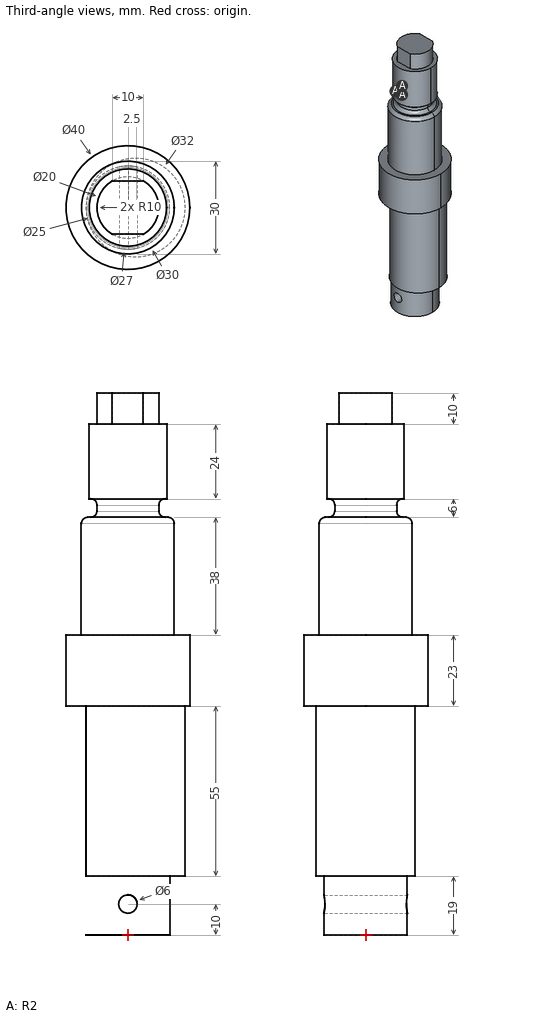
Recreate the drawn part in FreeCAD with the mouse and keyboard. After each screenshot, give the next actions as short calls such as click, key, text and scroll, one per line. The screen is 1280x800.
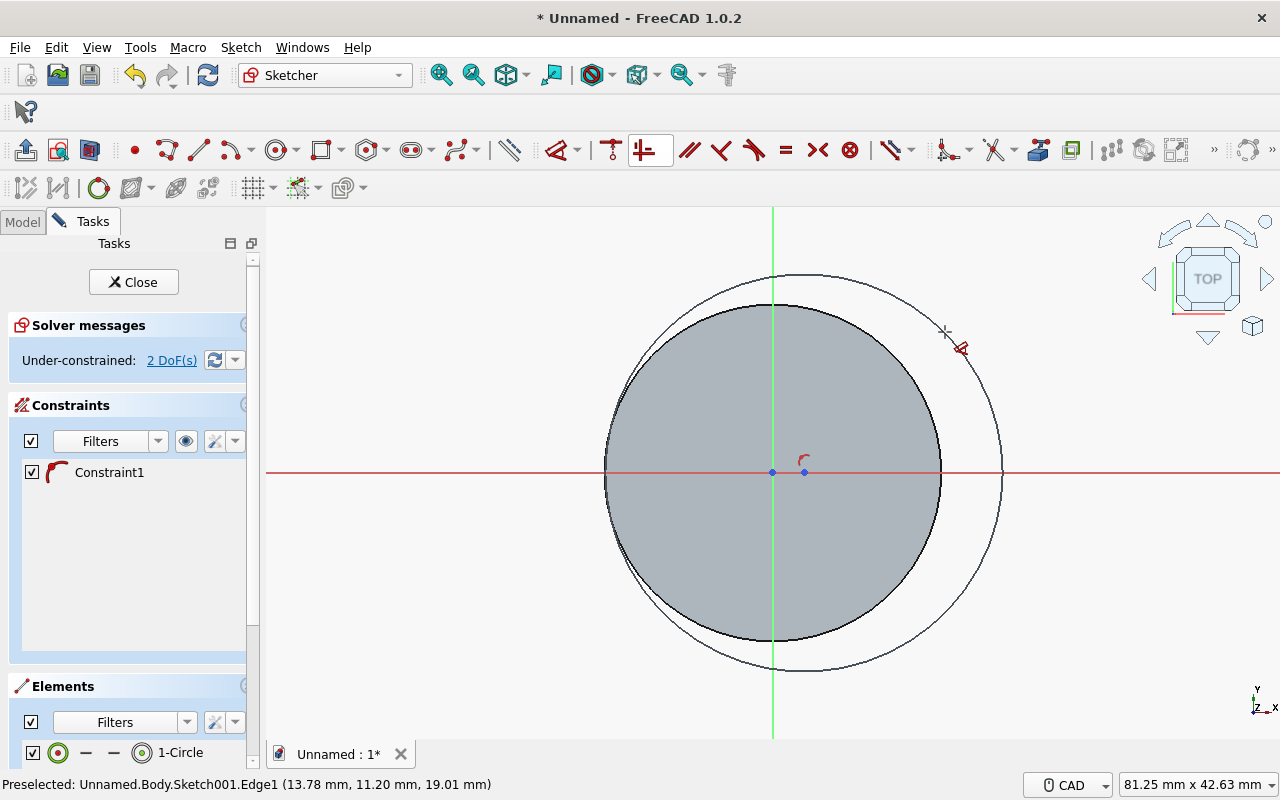
click(944, 332)
click(967, 309)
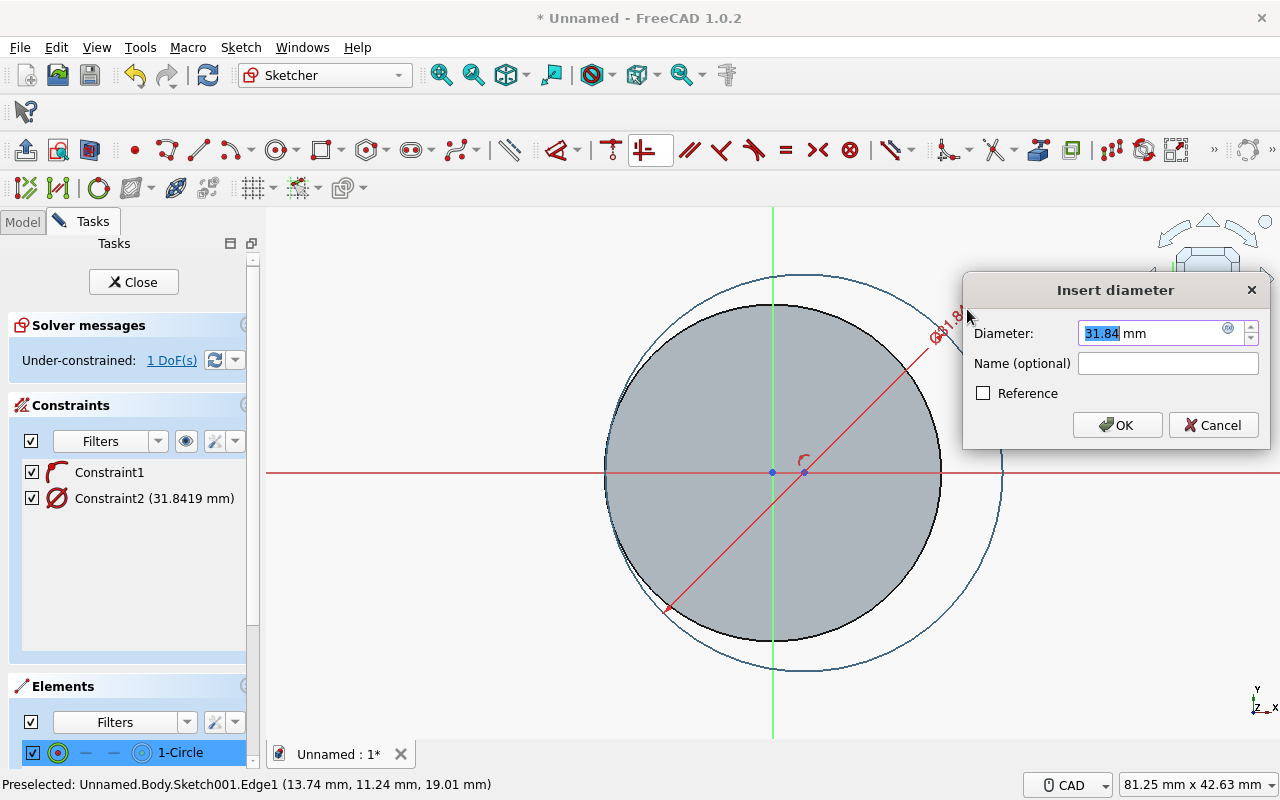
text(32)
key(Return)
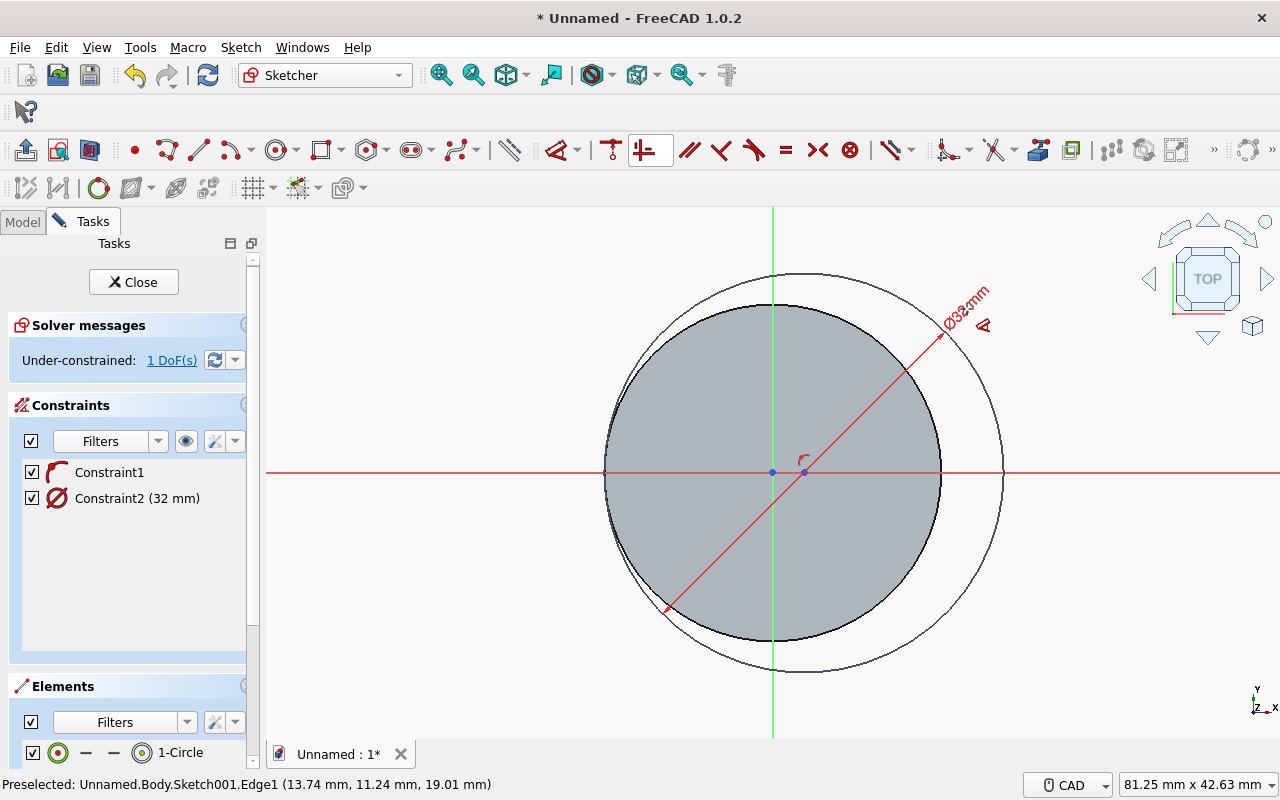
scroll(804, 473, up, 2)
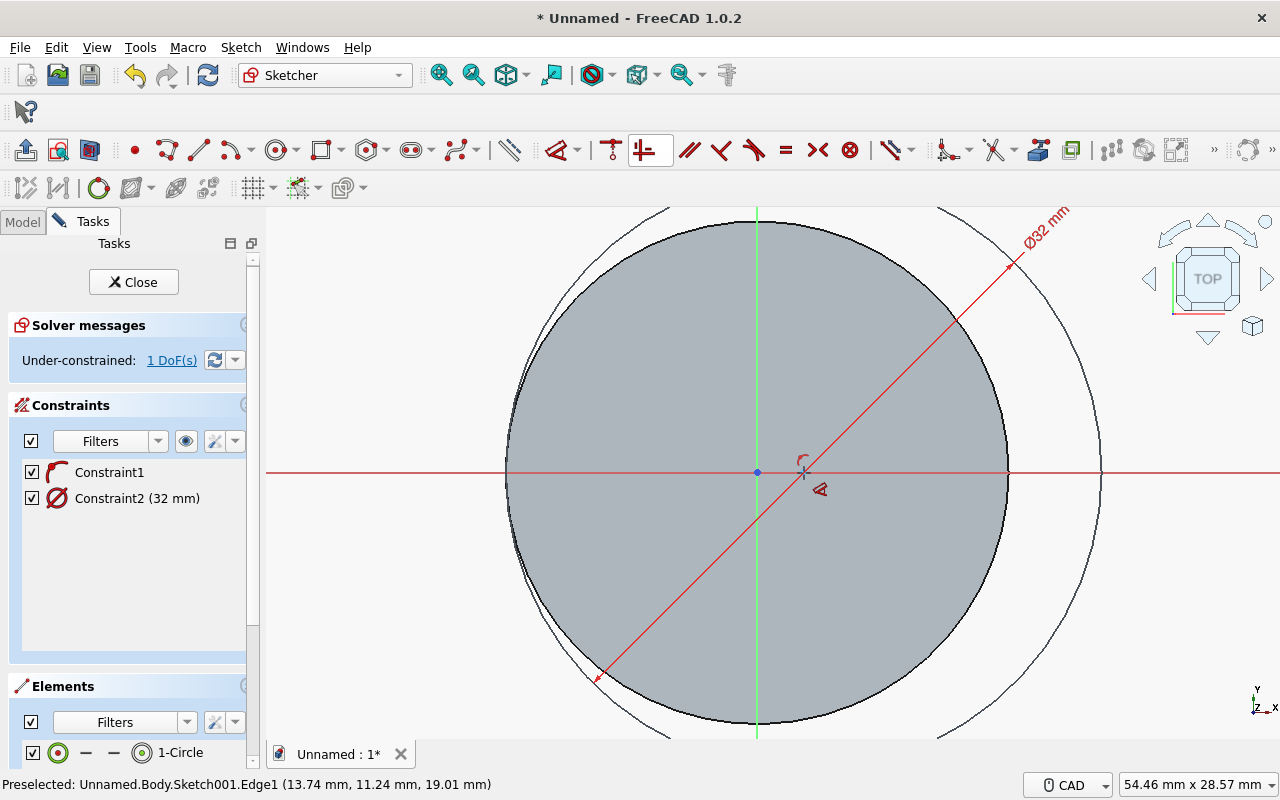
click(804, 473)
click(781, 507)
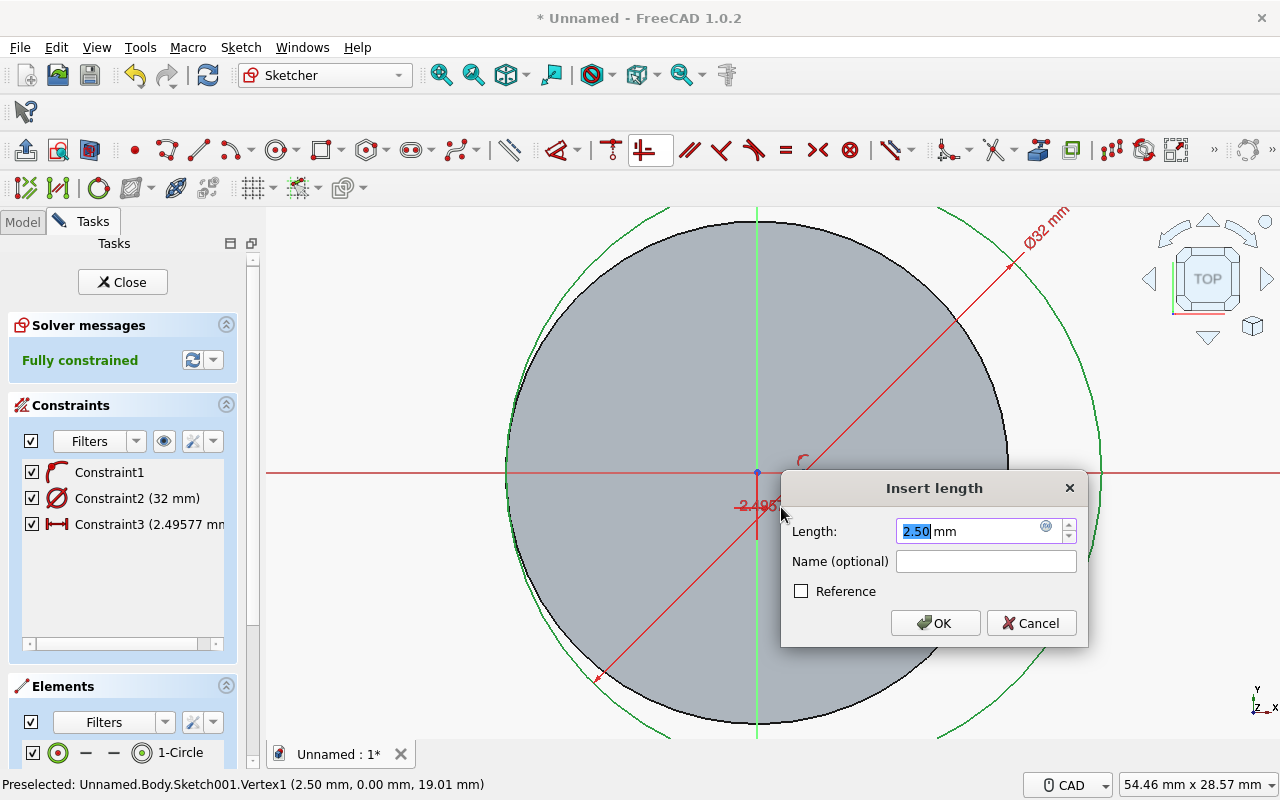
text(2.5)
key(Return)
key(Escape)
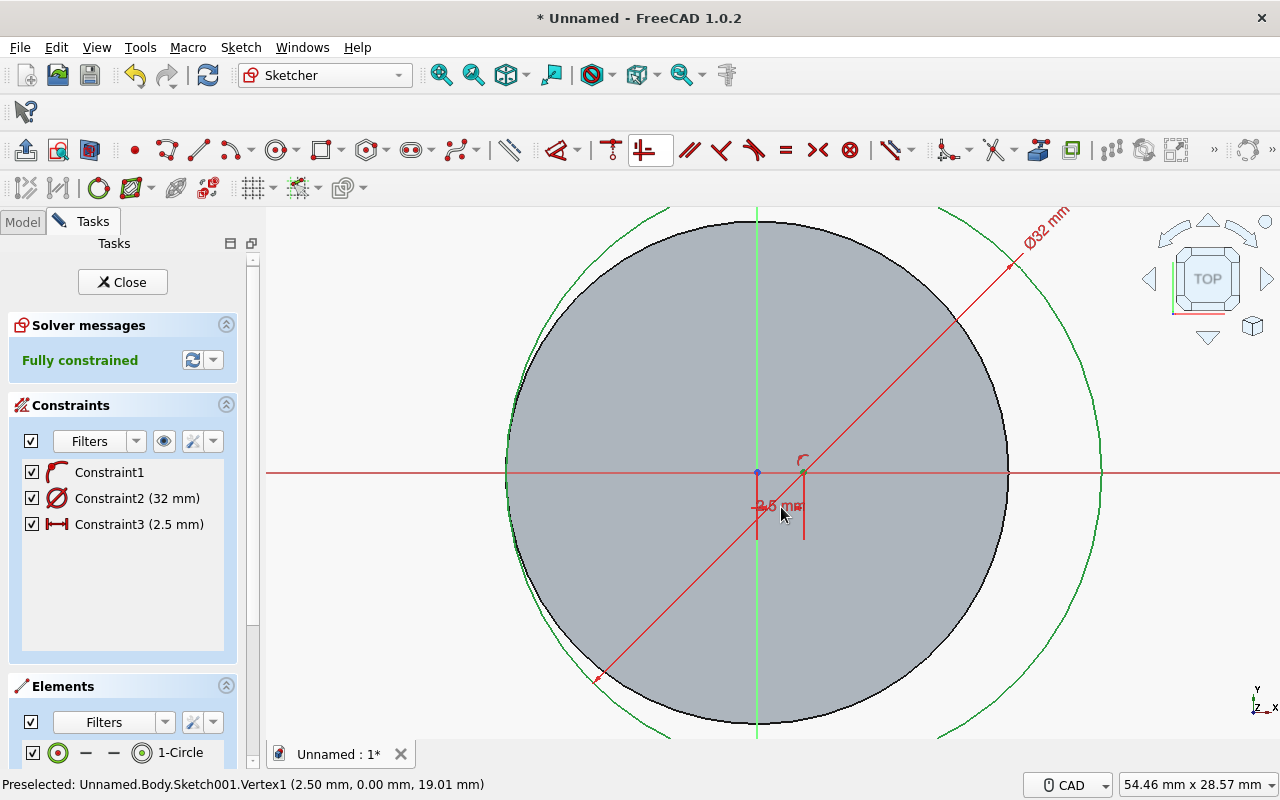
click(123, 282)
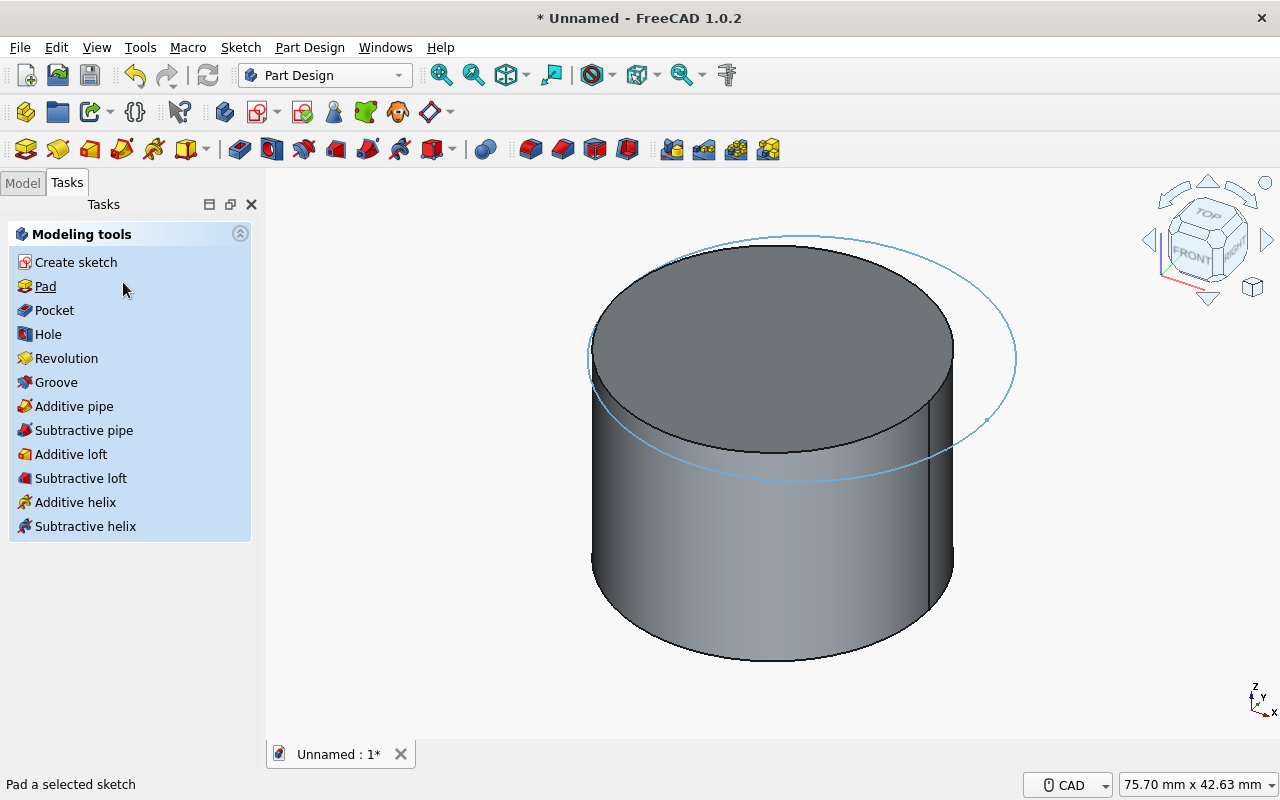
click(26, 150)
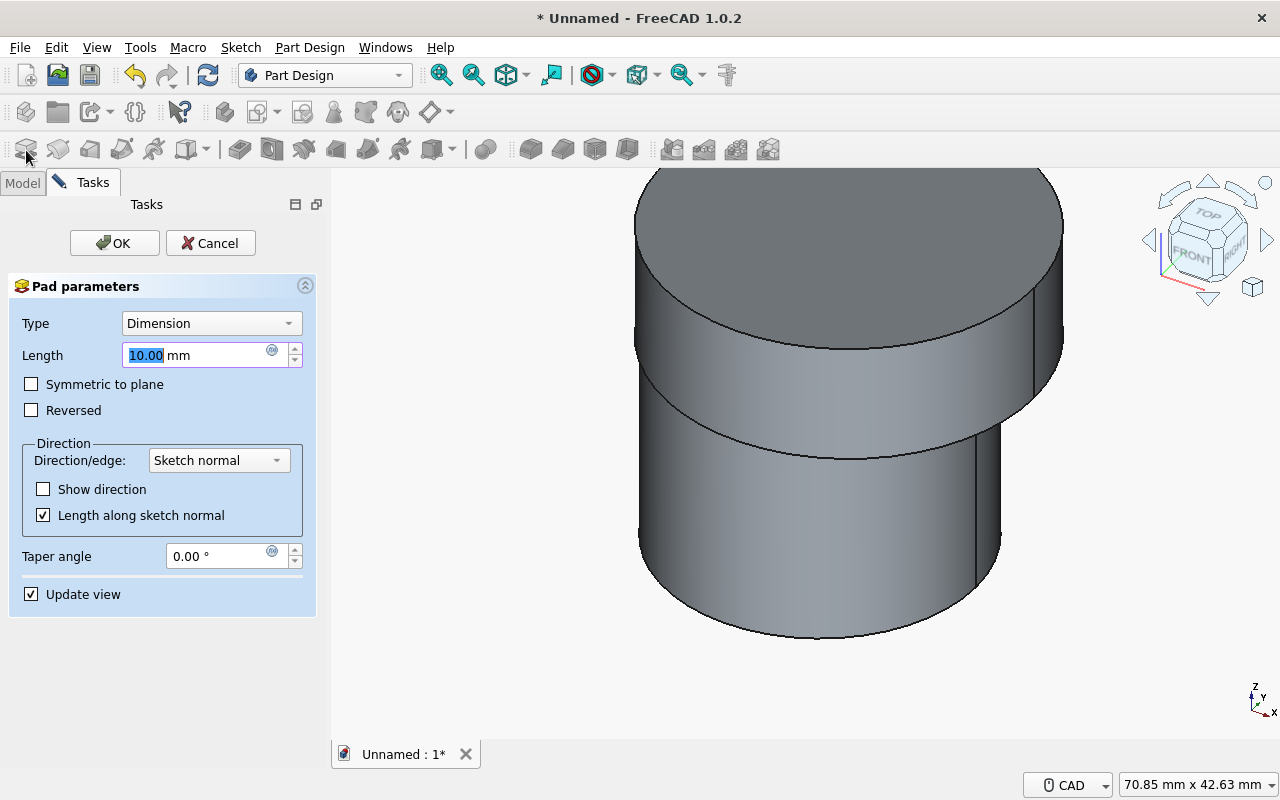
text(55)
key(Tab)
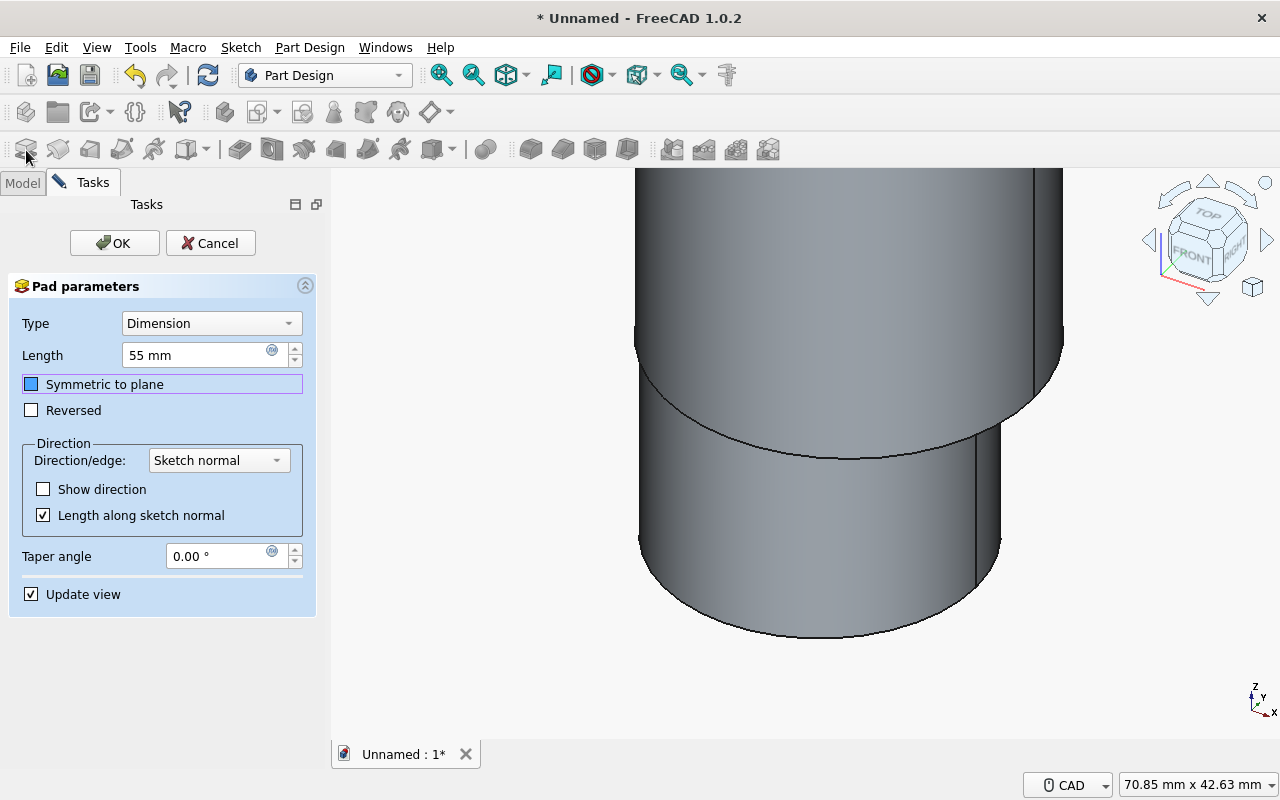
click(115, 243)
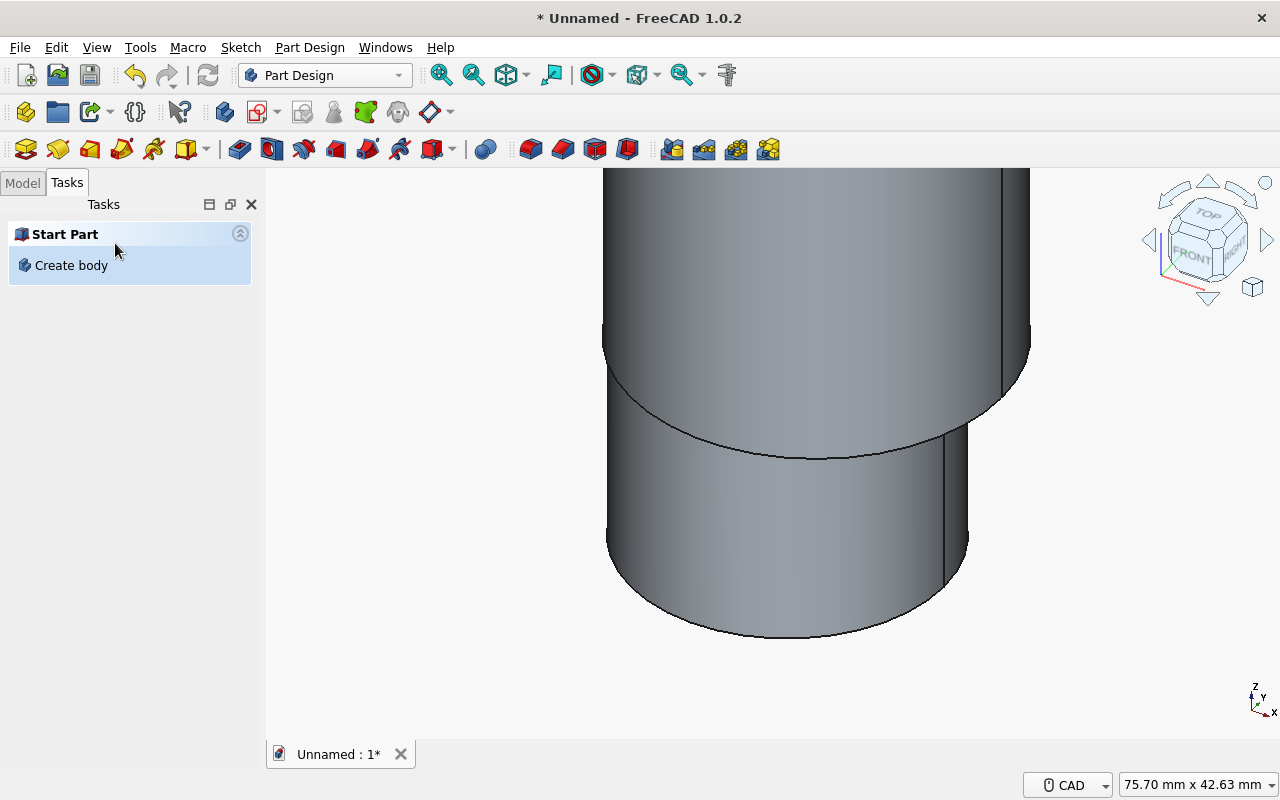
key(v)
key(f)